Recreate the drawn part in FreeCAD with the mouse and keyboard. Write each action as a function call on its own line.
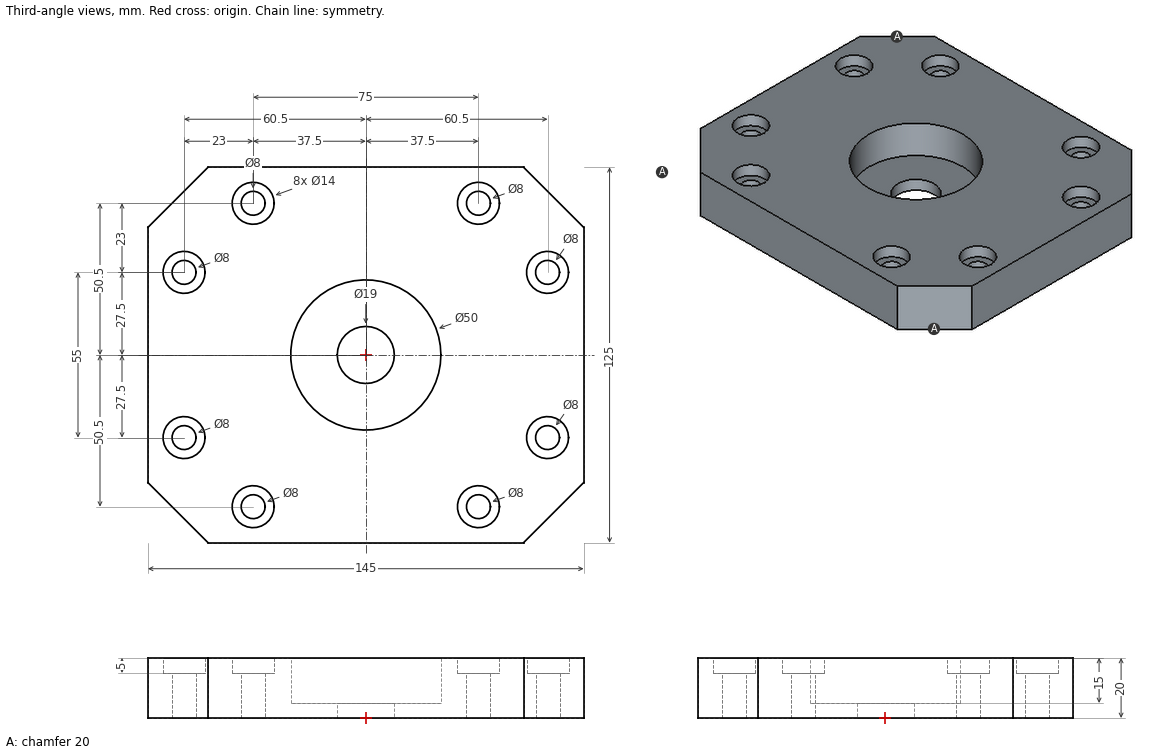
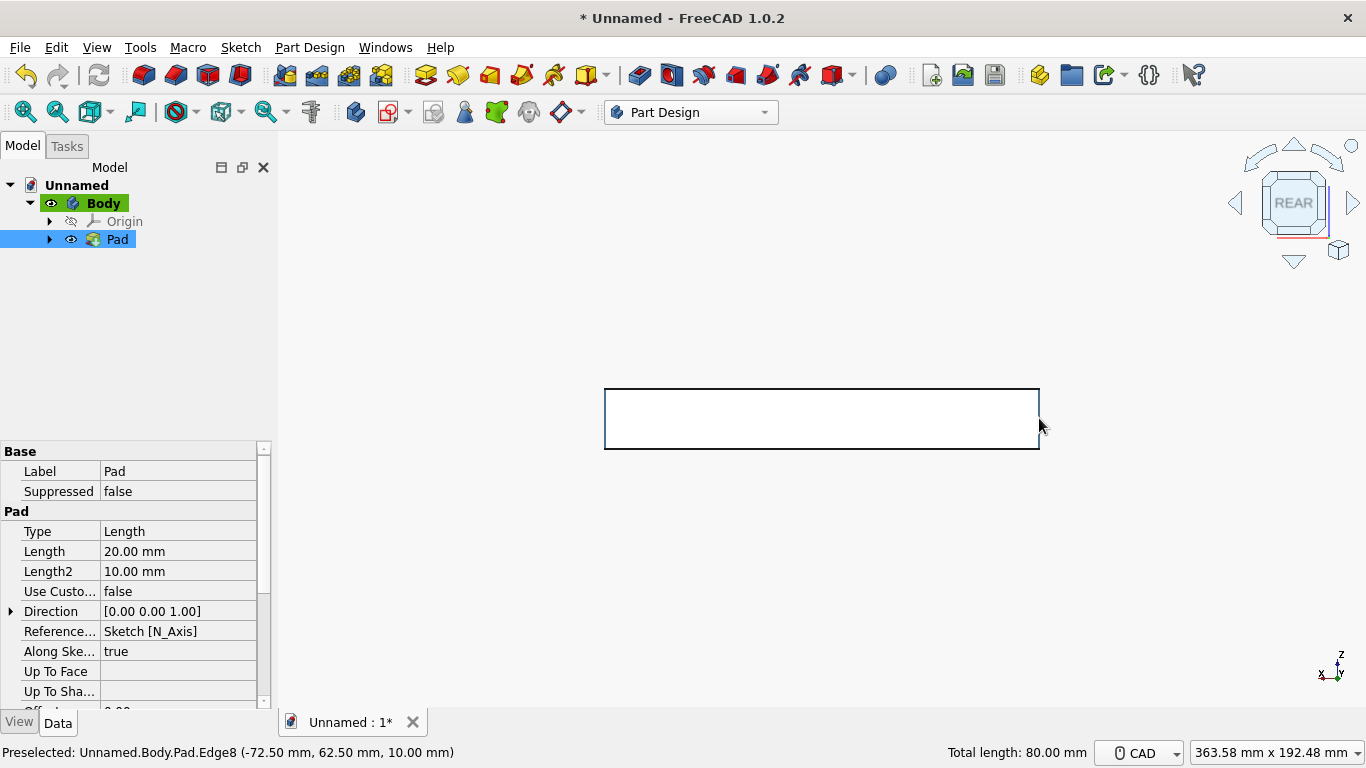
click(176, 76)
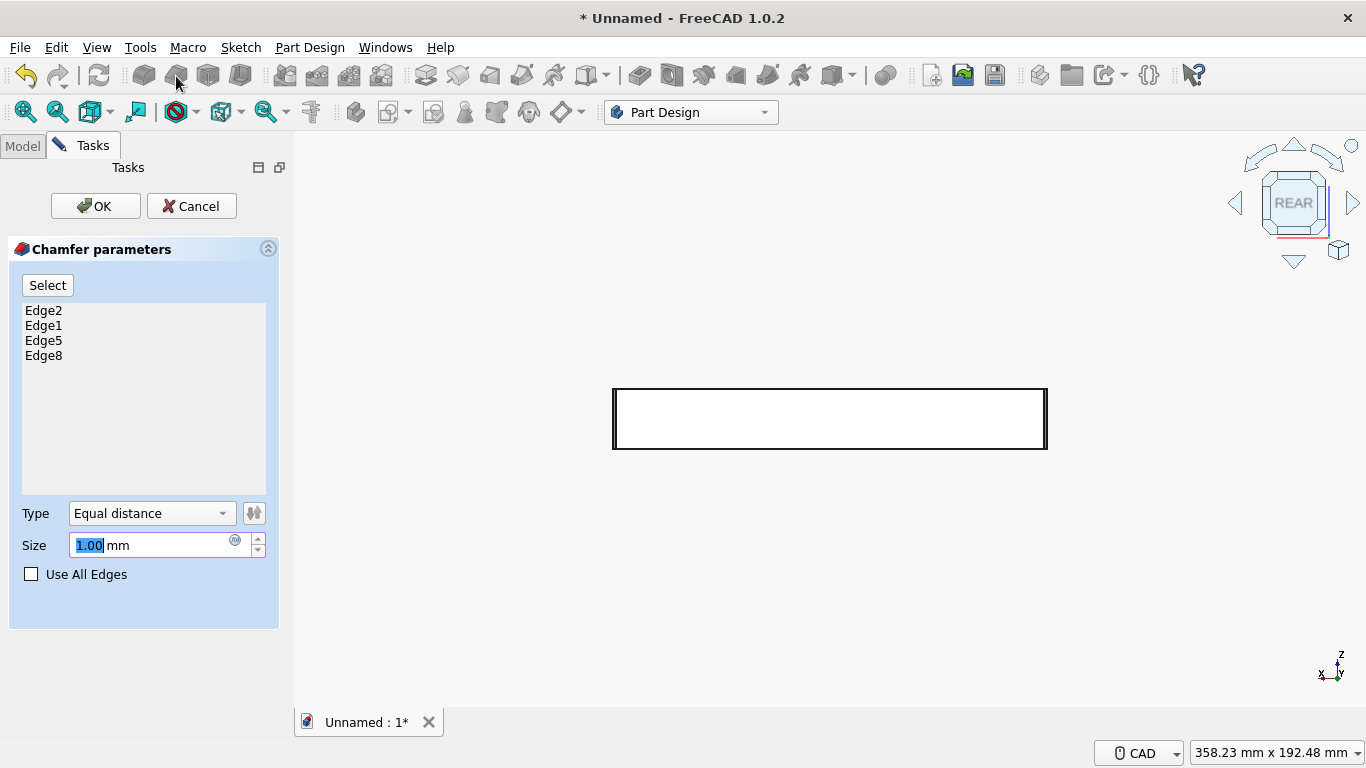
text(20)
key(Tab)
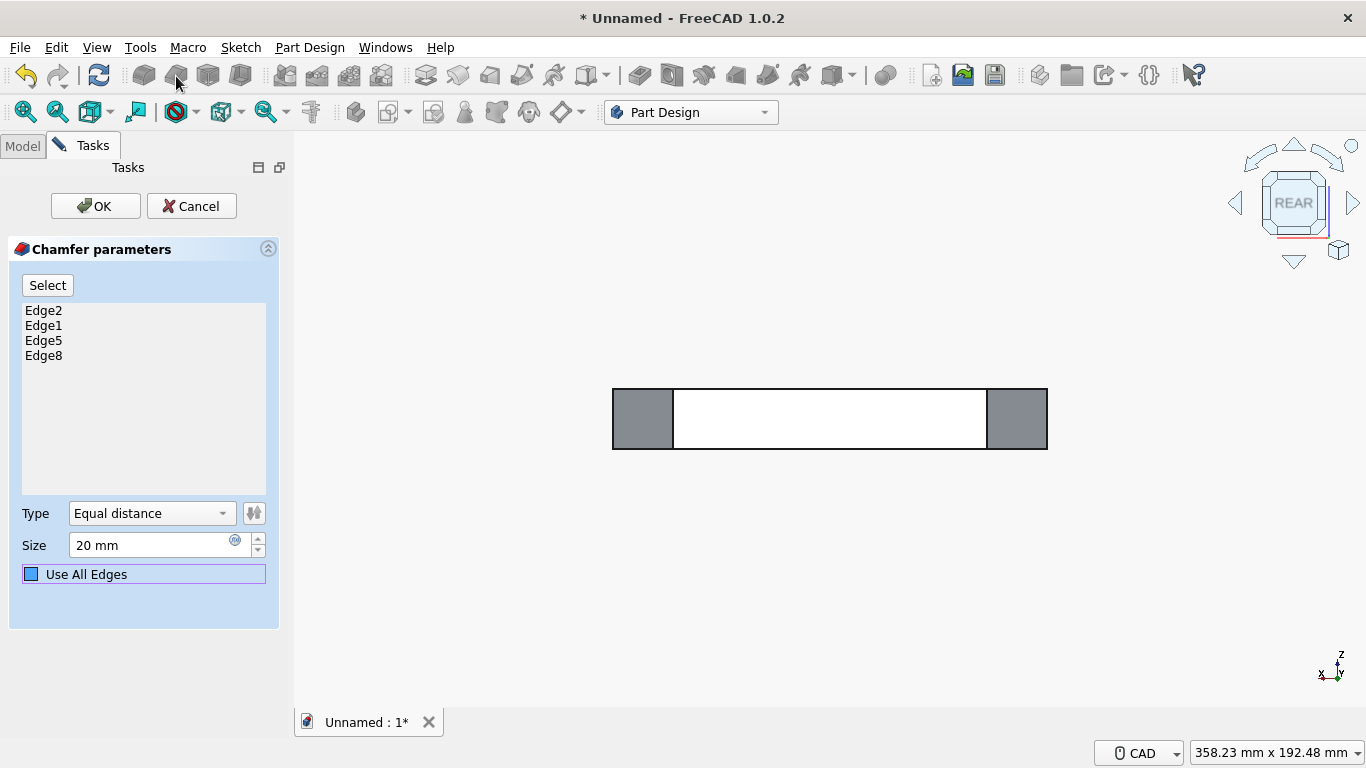
click(96, 206)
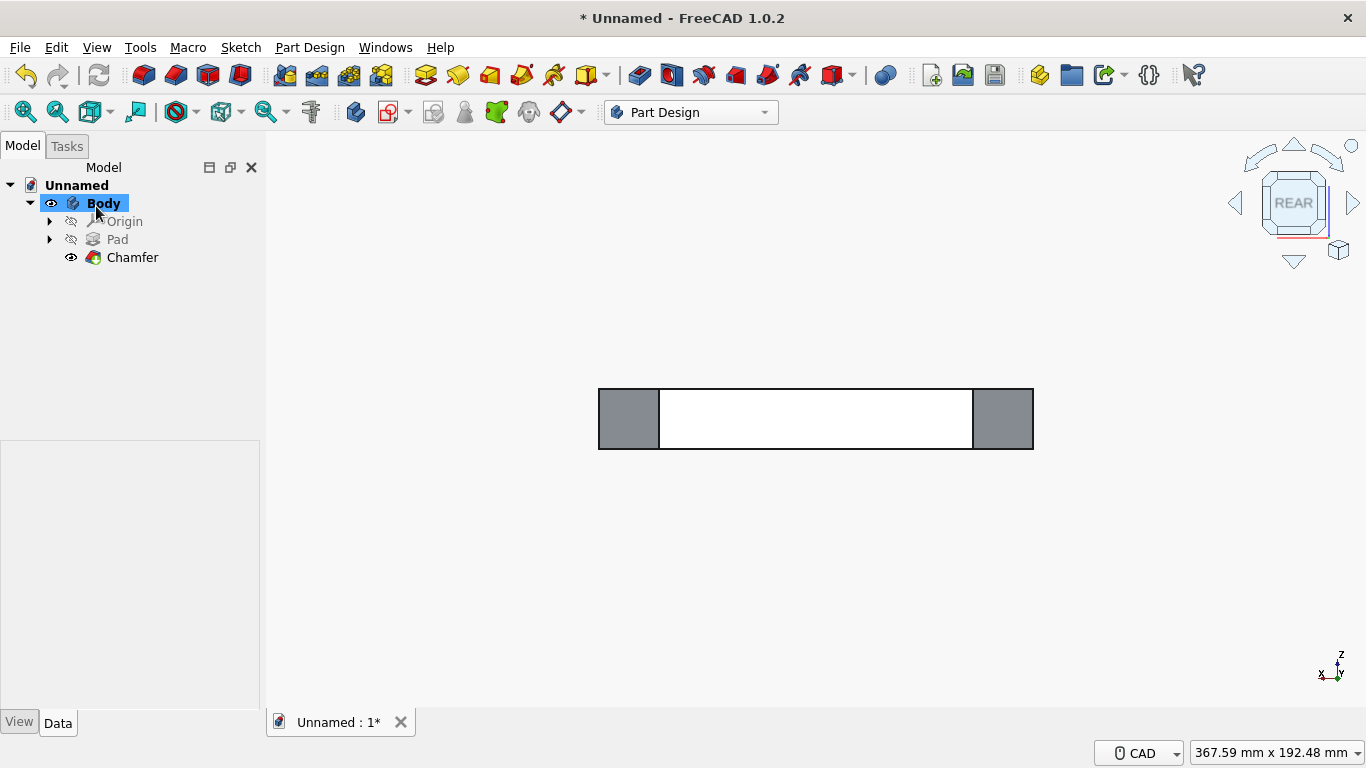
click(26, 112)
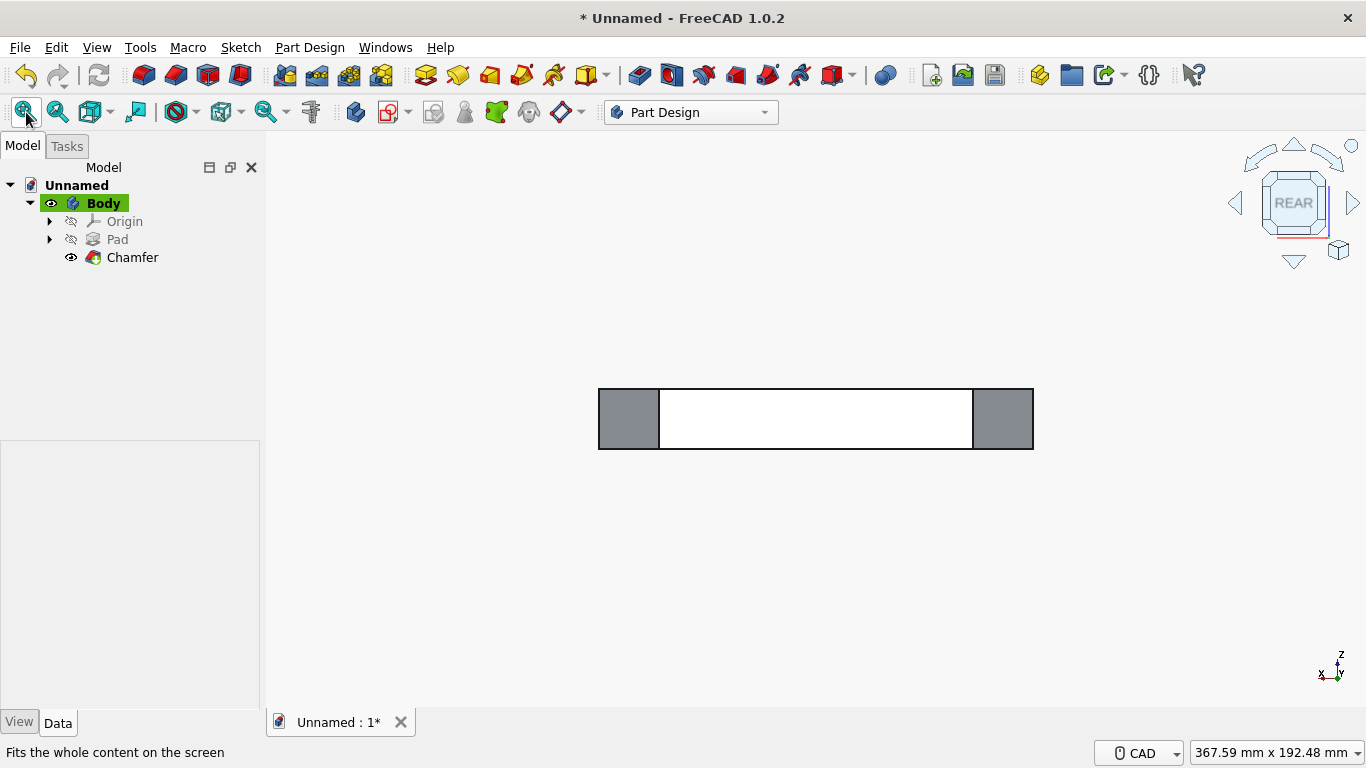
key(0)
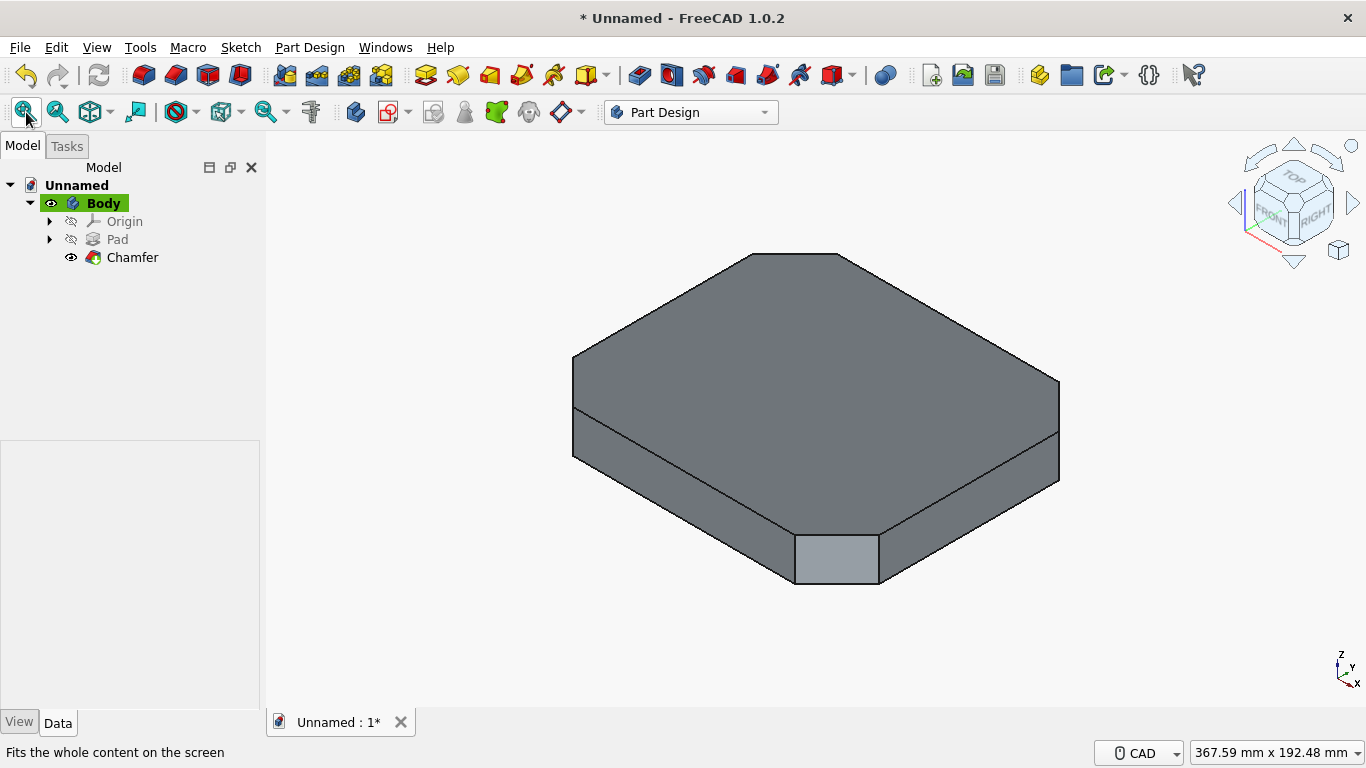
click(816, 394)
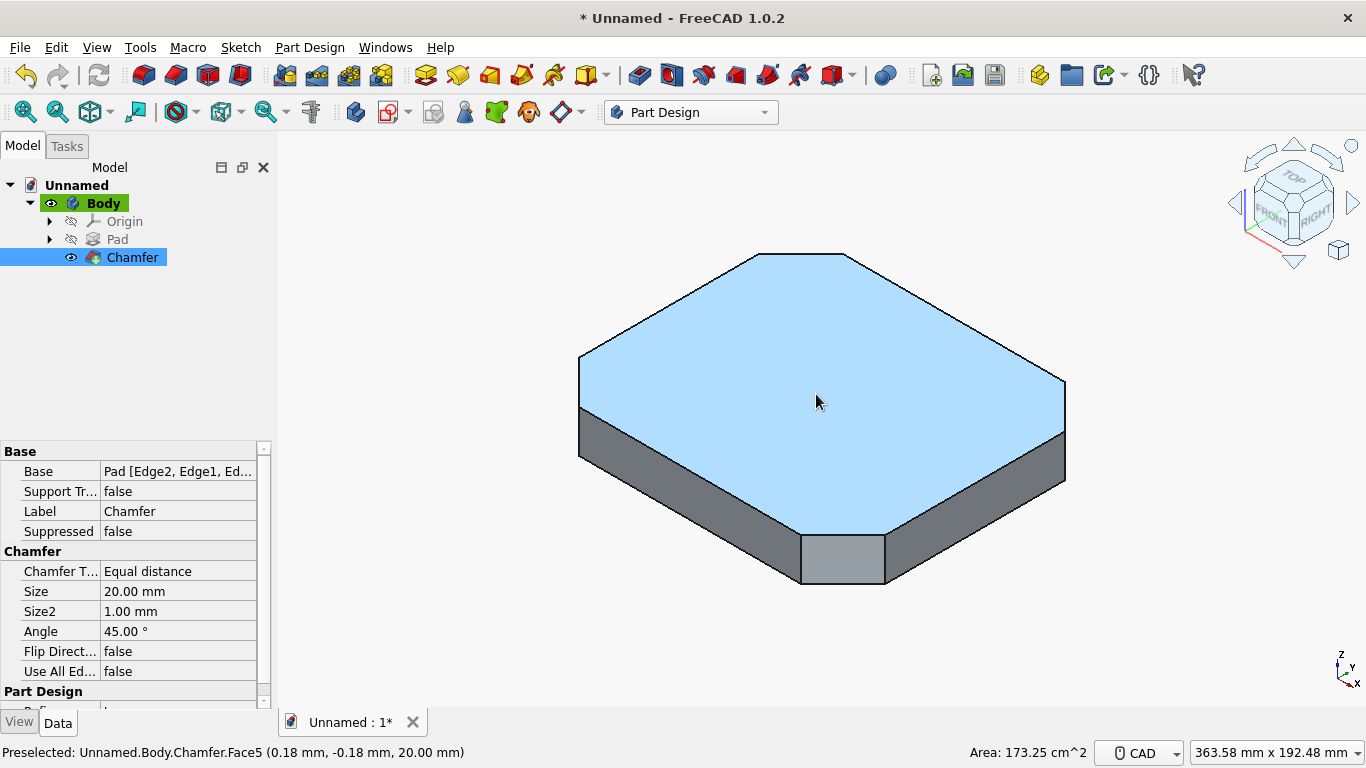
click(388, 112)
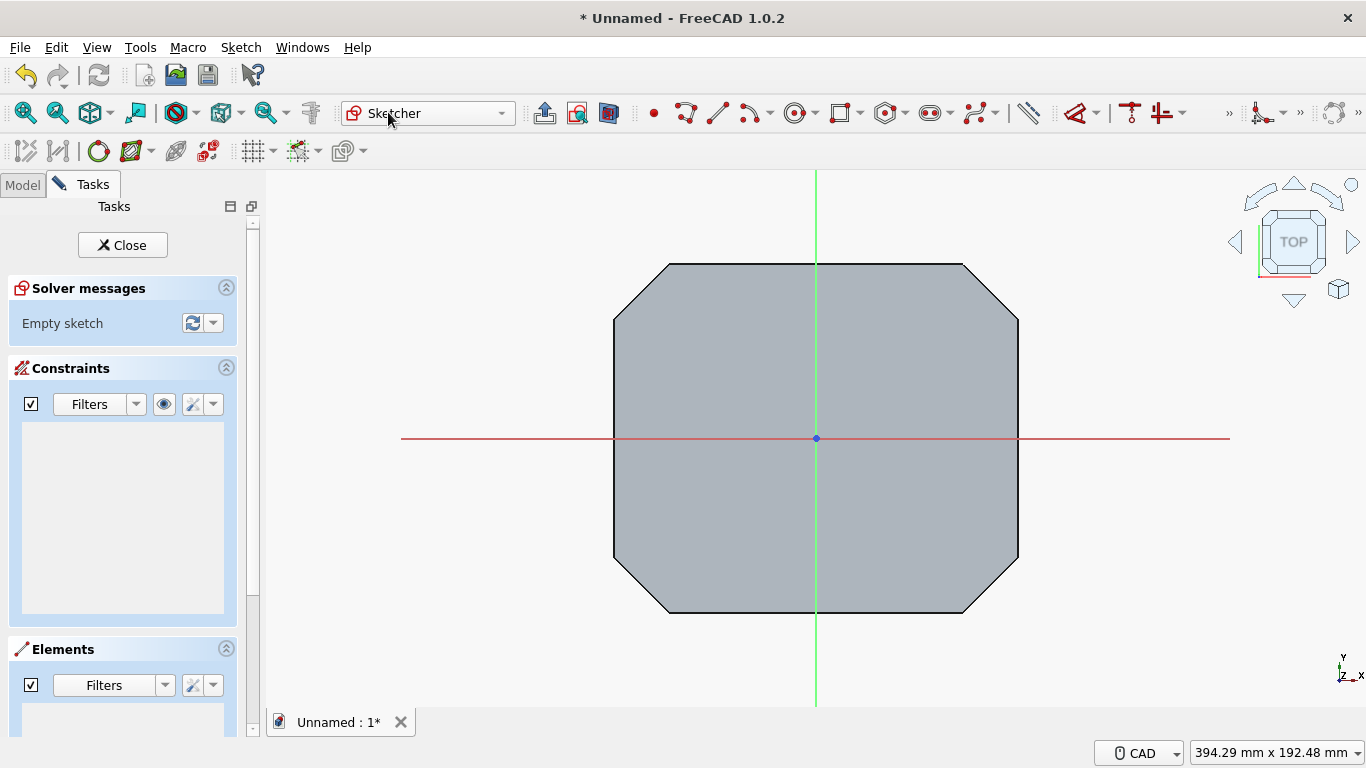
click(796, 114)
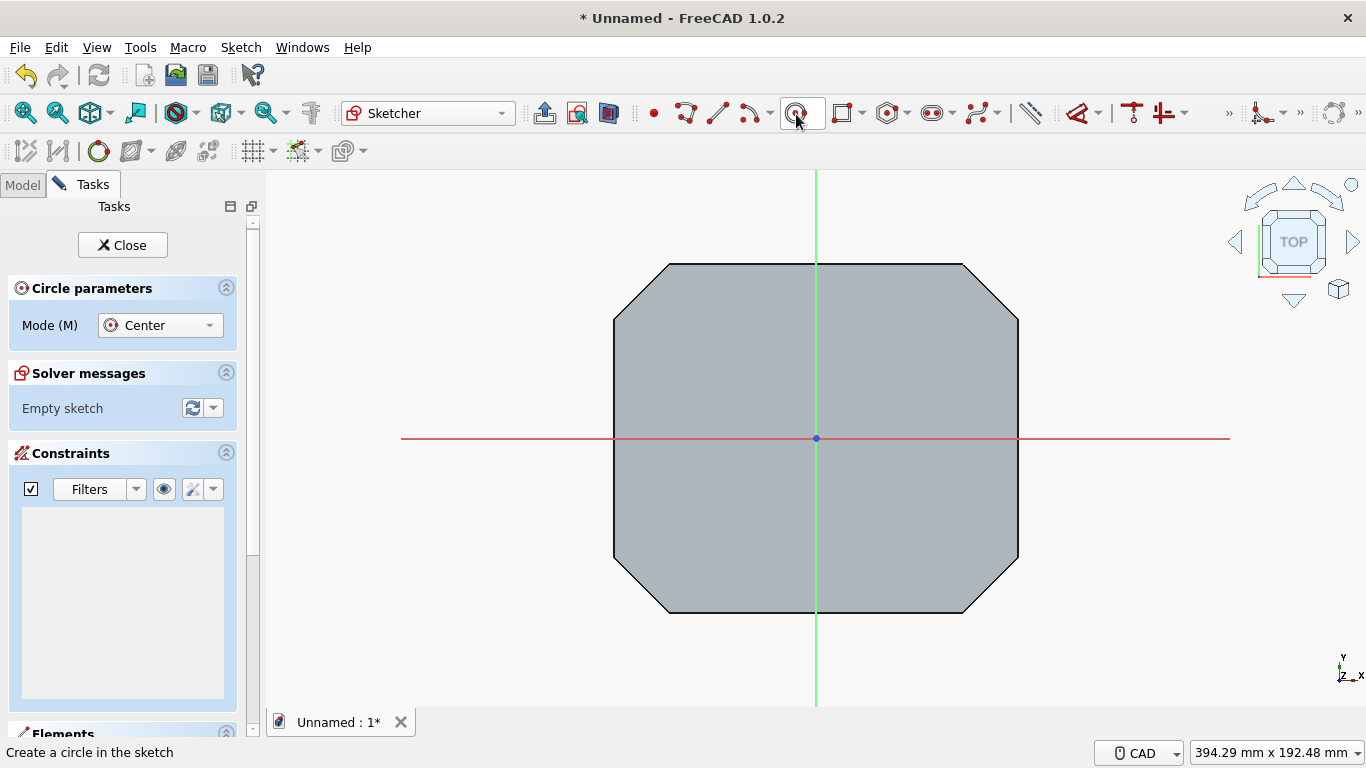
click(711, 298)
click(725, 284)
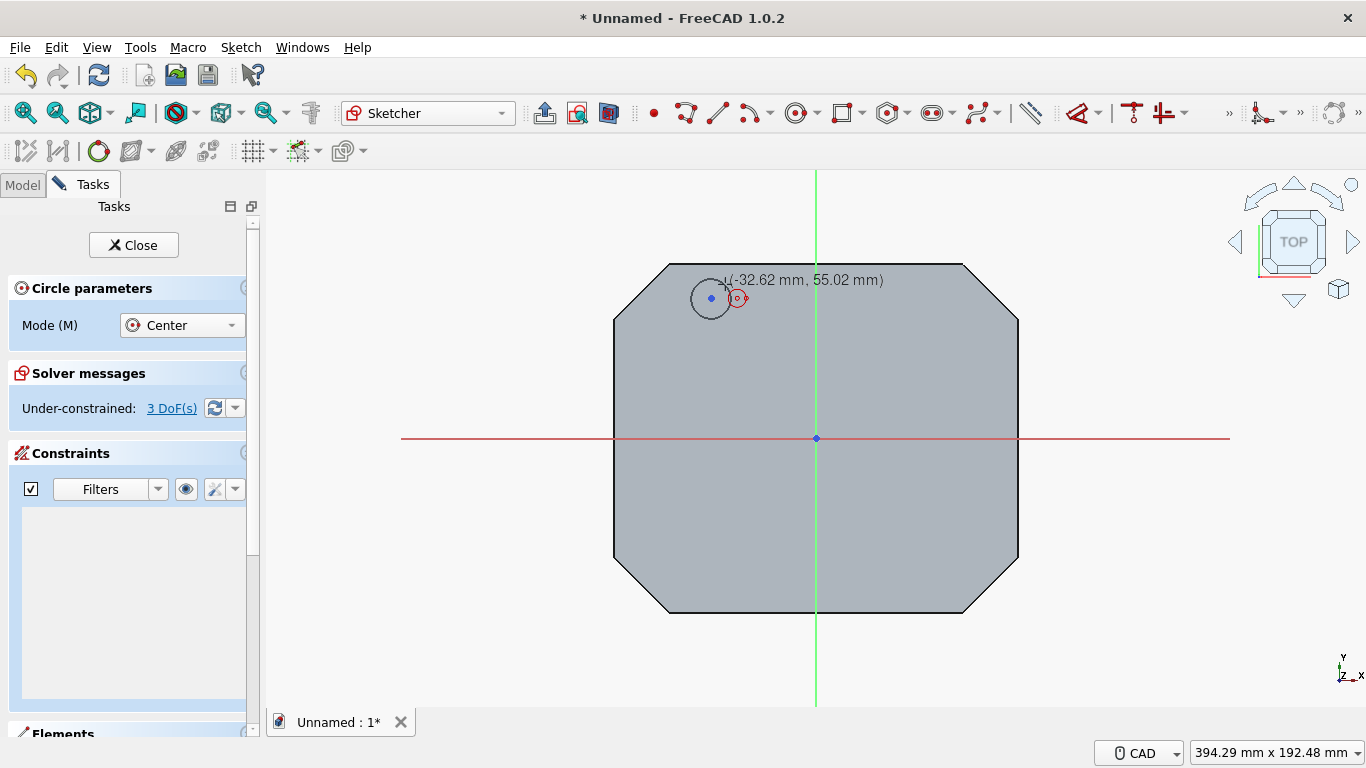
click(921, 298)
click(934, 284)